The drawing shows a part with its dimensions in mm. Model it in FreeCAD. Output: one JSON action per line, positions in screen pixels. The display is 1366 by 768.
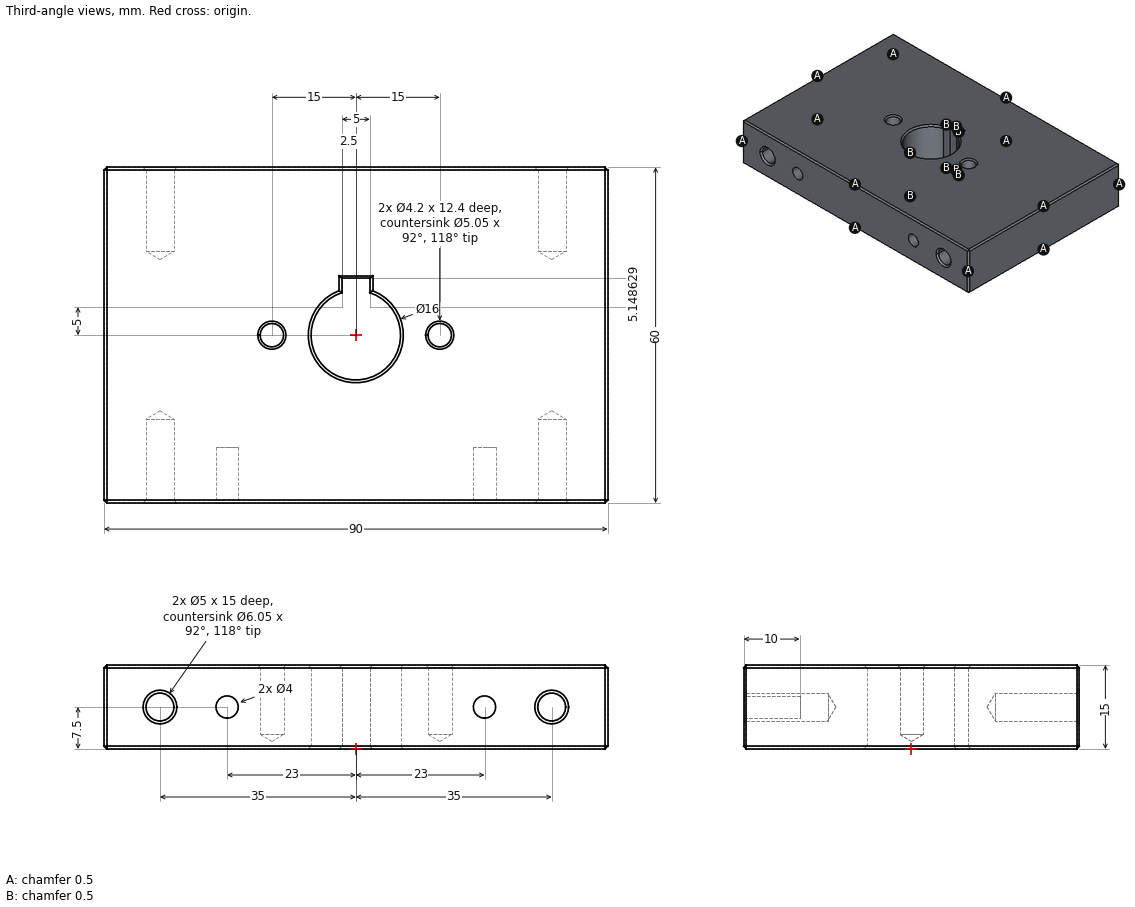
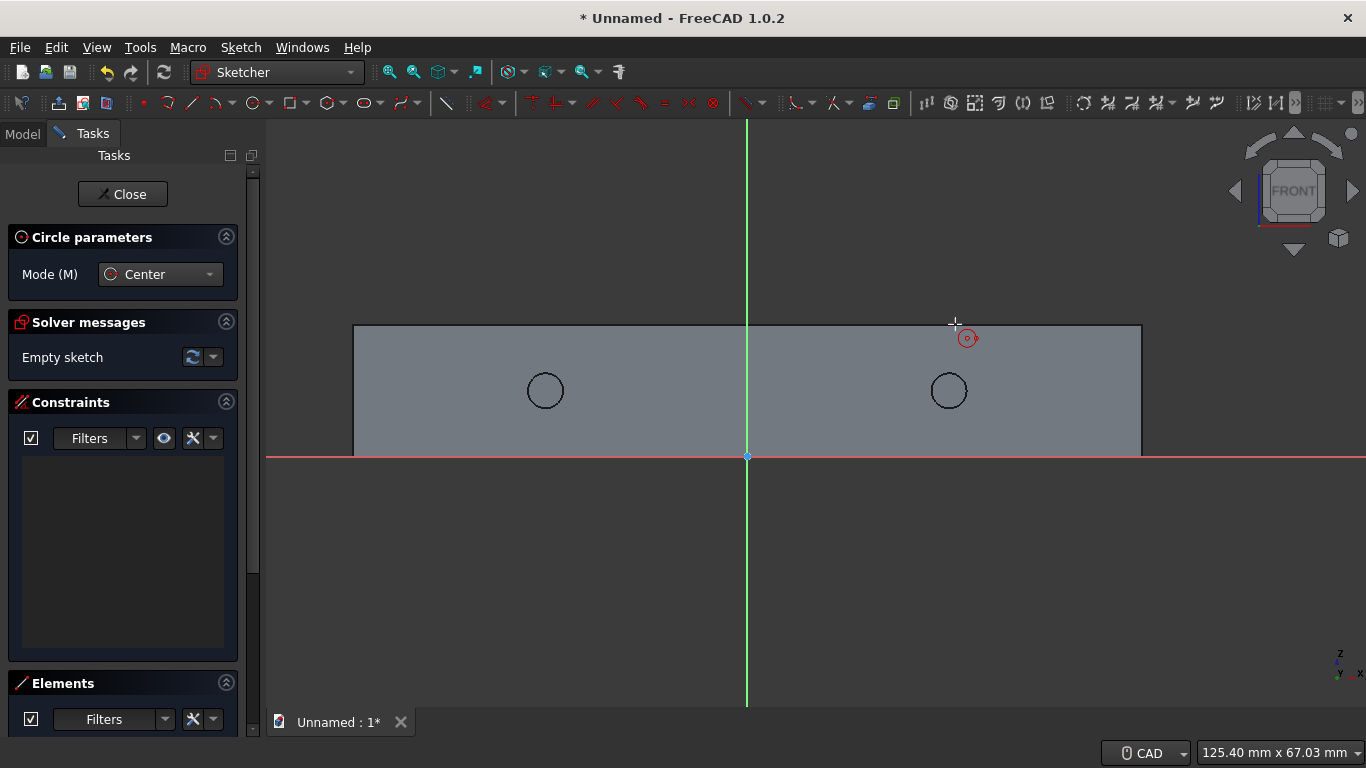
{"action": "left_click", "coordinate": [440, 391]}
{"action": "mouse_move", "coordinate": [456, 375]}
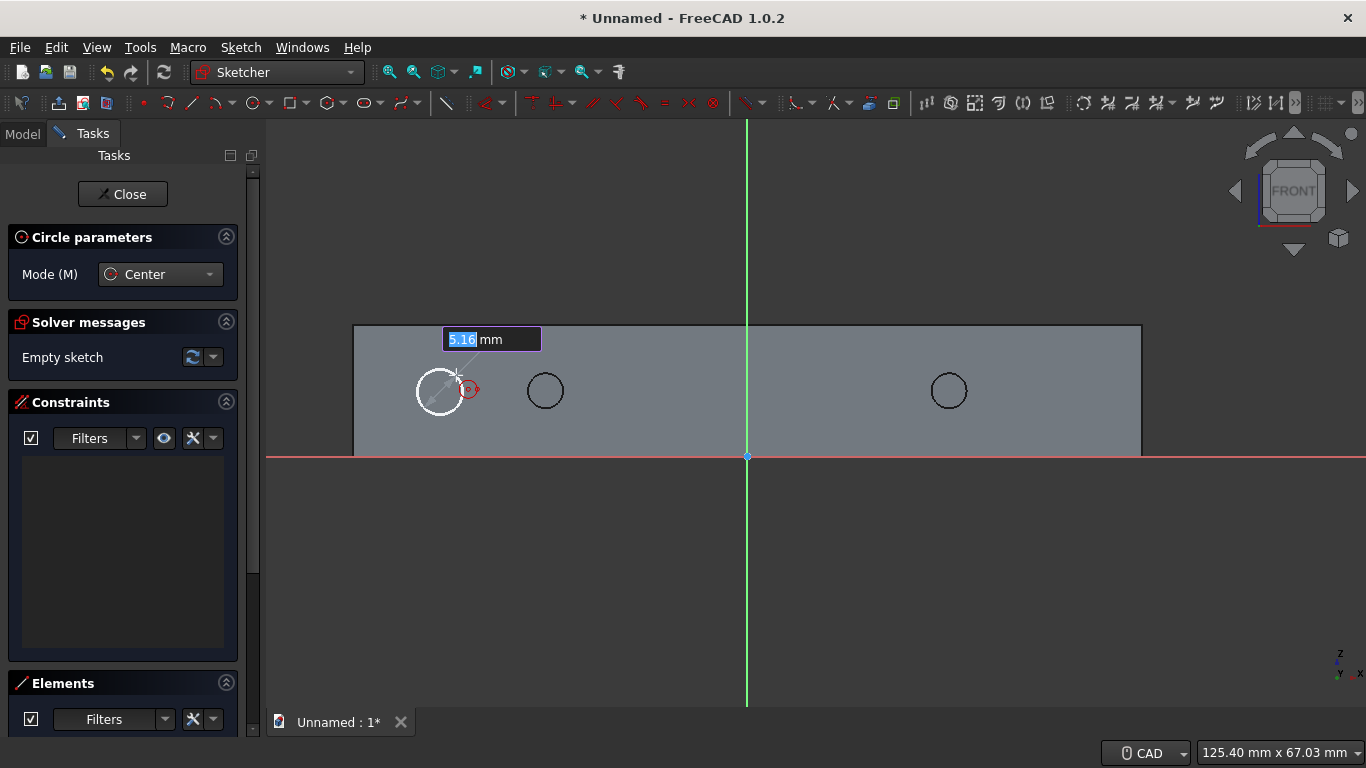
{"action": "type", "text": "5"}
{"action": "key", "text": "Return"}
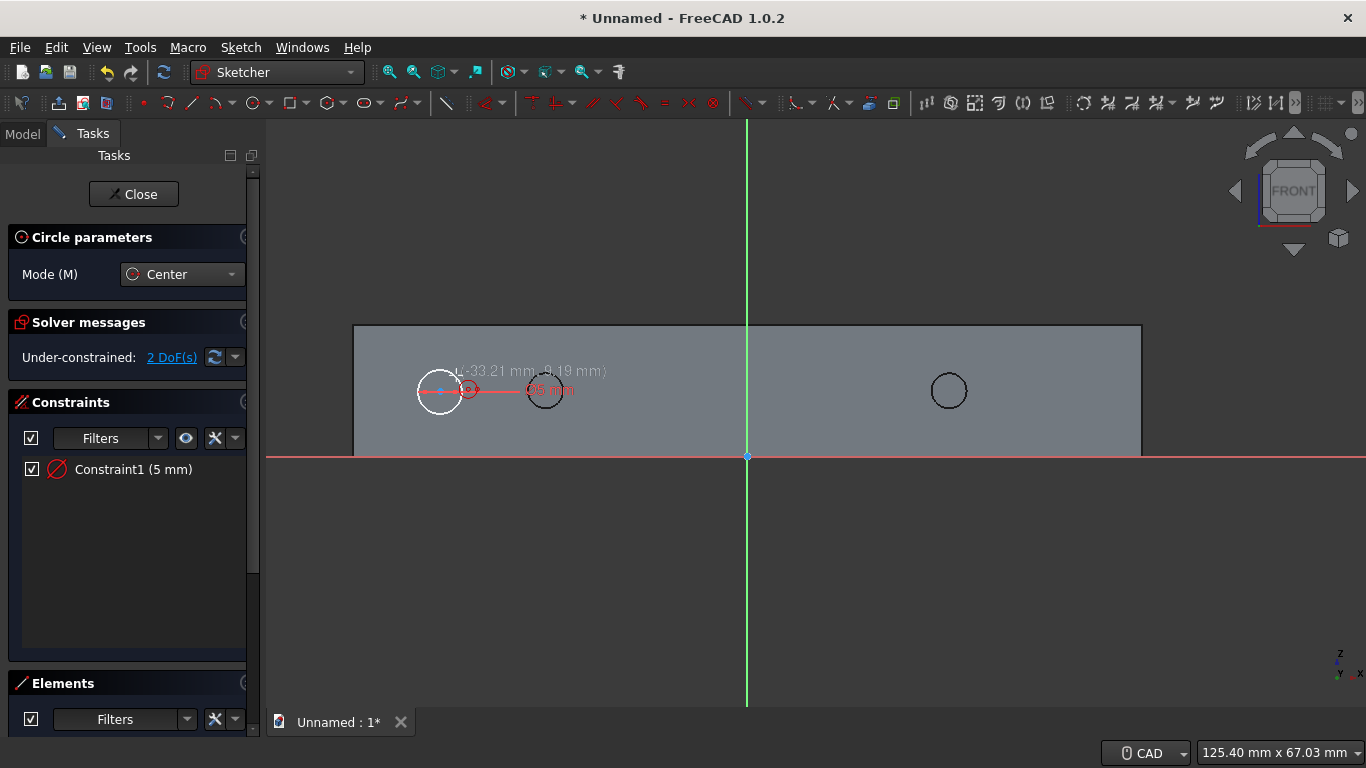
{"action": "left_click", "coordinate": [1054, 391]}
{"action": "mouse_move", "coordinate": [1070, 375]}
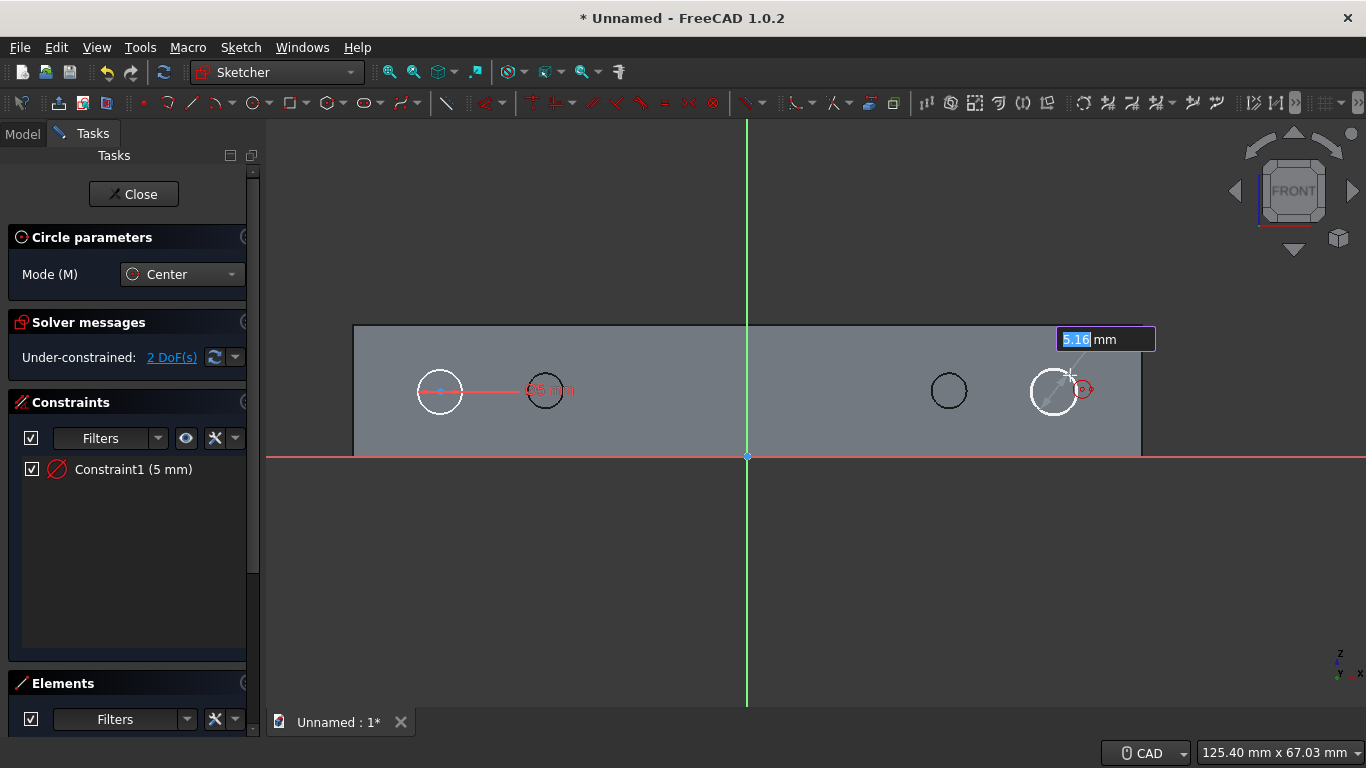
{"action": "type", "text": "5"}
{"action": "key", "text": "Return"}
{"action": "key", "text": "Escape"}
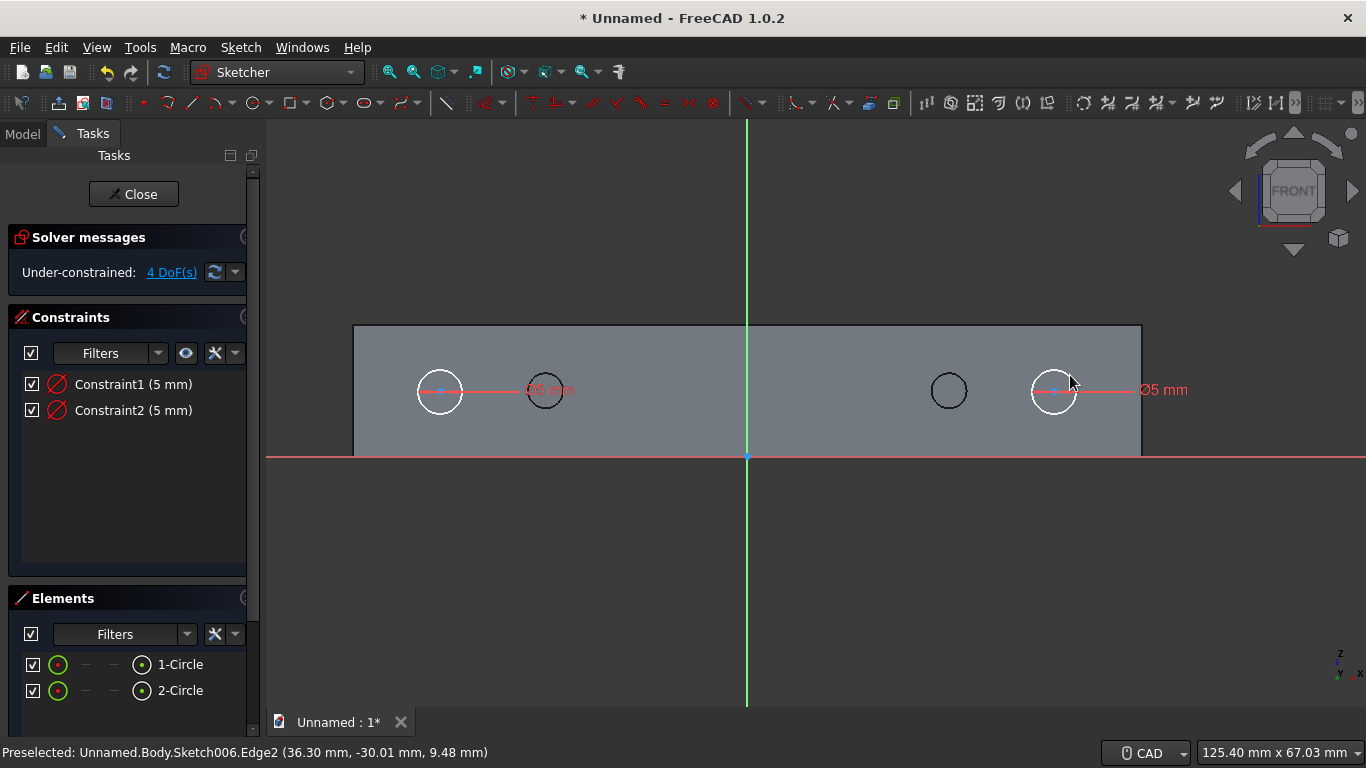
{"action": "left_click", "coordinate": [440, 392]}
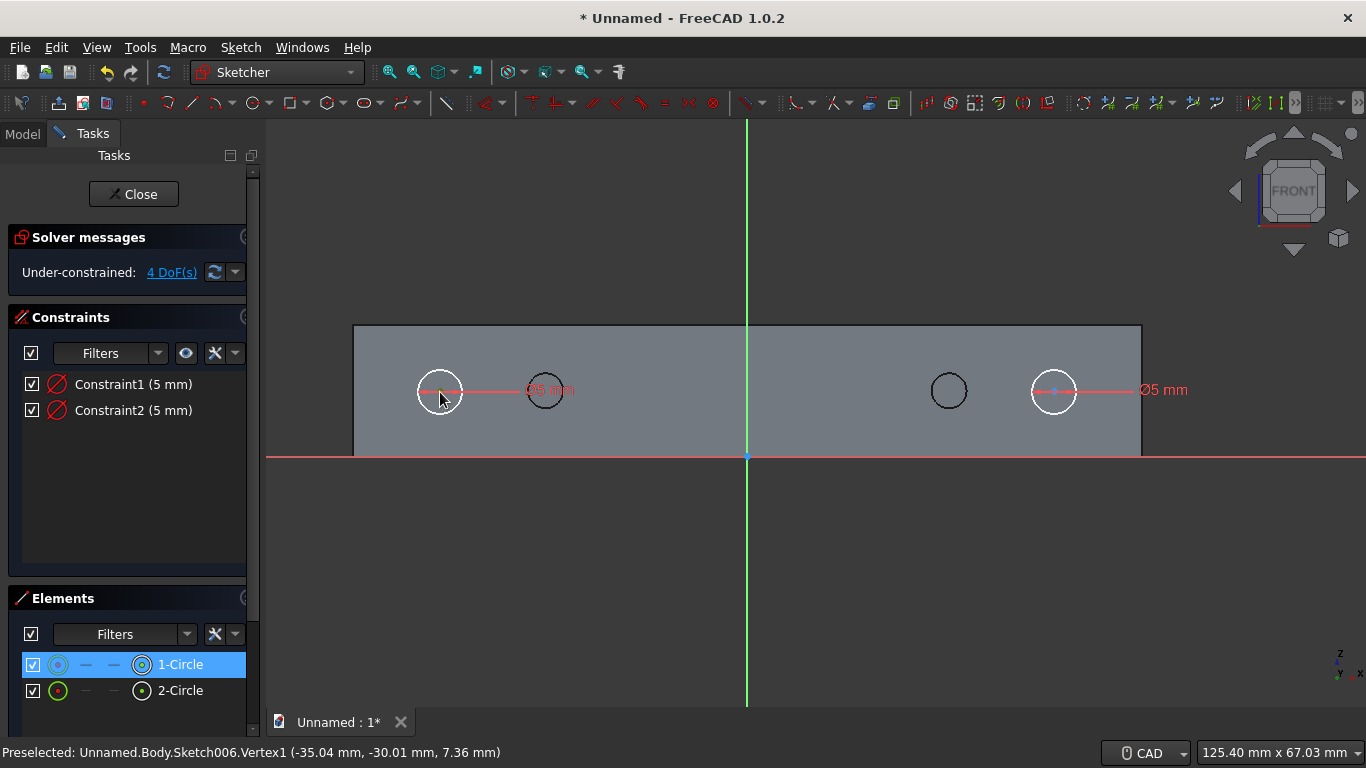
{"action": "left_click", "coordinate": [1054, 392]}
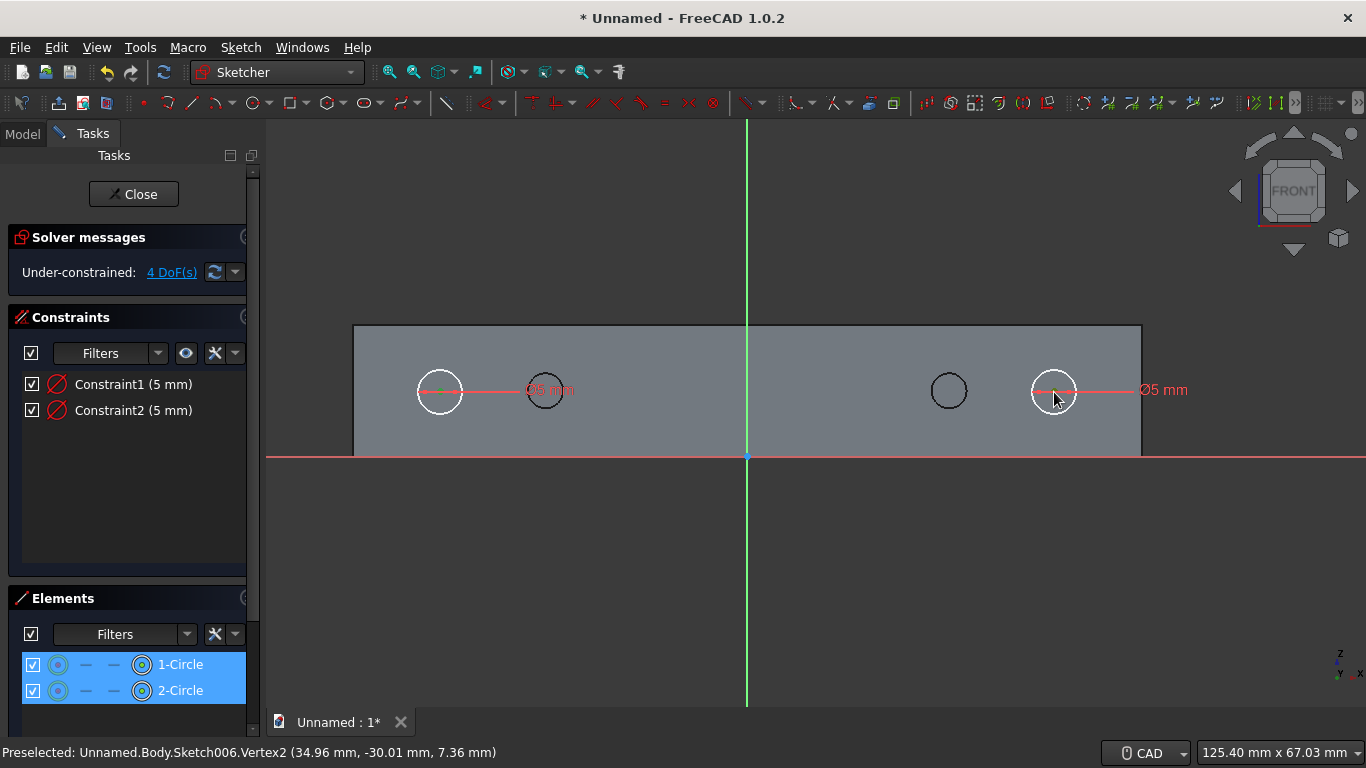
{"action": "key", "text": "h"}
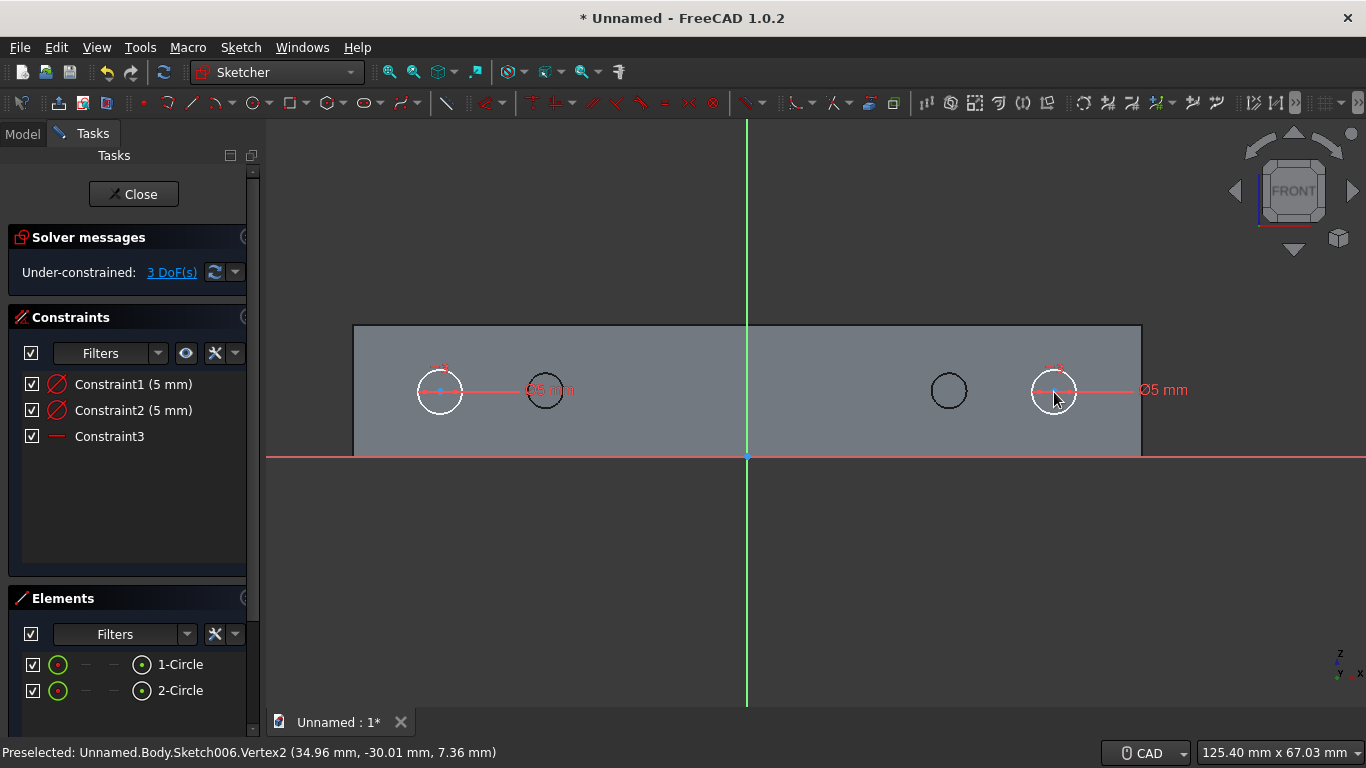
{"action": "left_click", "coordinate": [486, 104]}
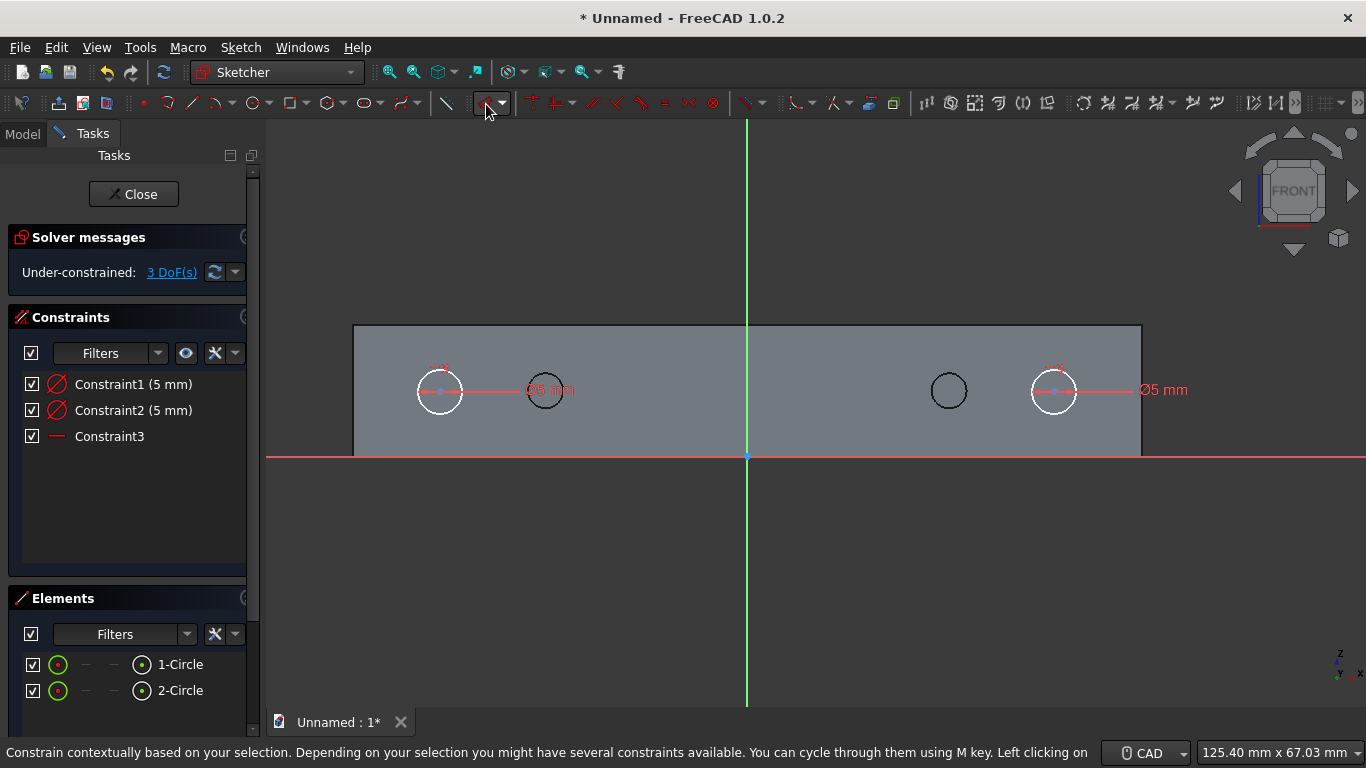
{"action": "left_click", "coordinate": [440, 392]}
{"action": "left_click", "coordinate": [594, 491]}